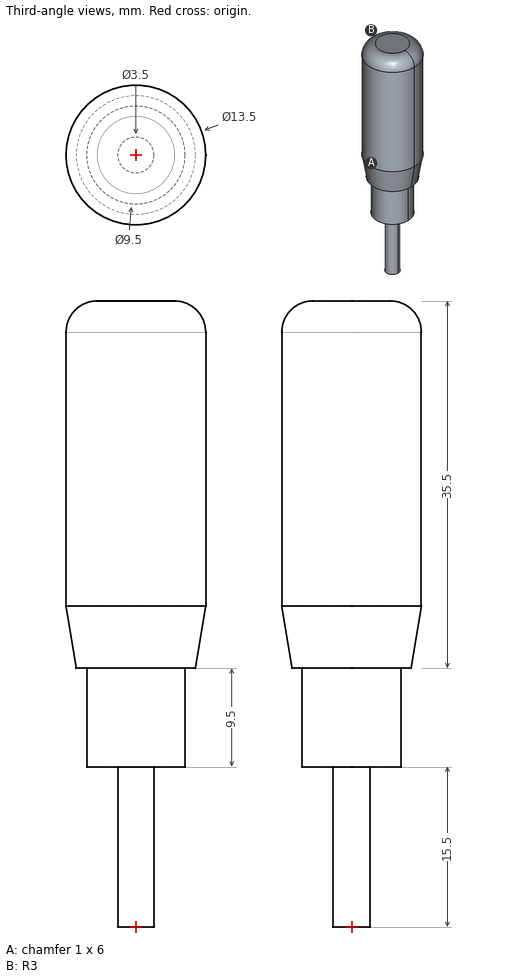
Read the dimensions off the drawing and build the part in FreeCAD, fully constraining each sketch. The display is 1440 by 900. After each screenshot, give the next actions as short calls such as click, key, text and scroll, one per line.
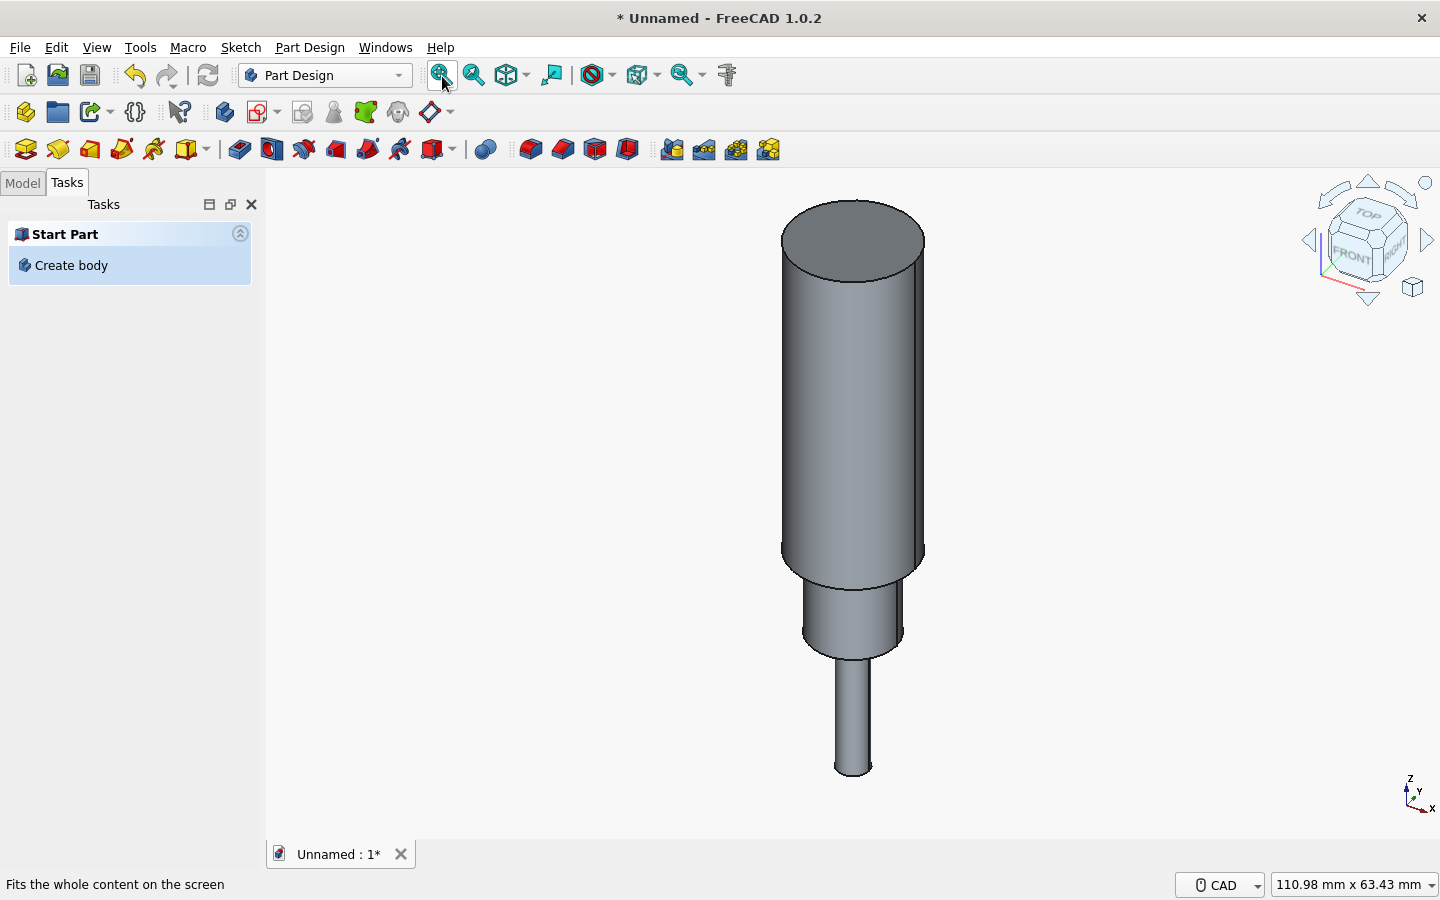
key(0)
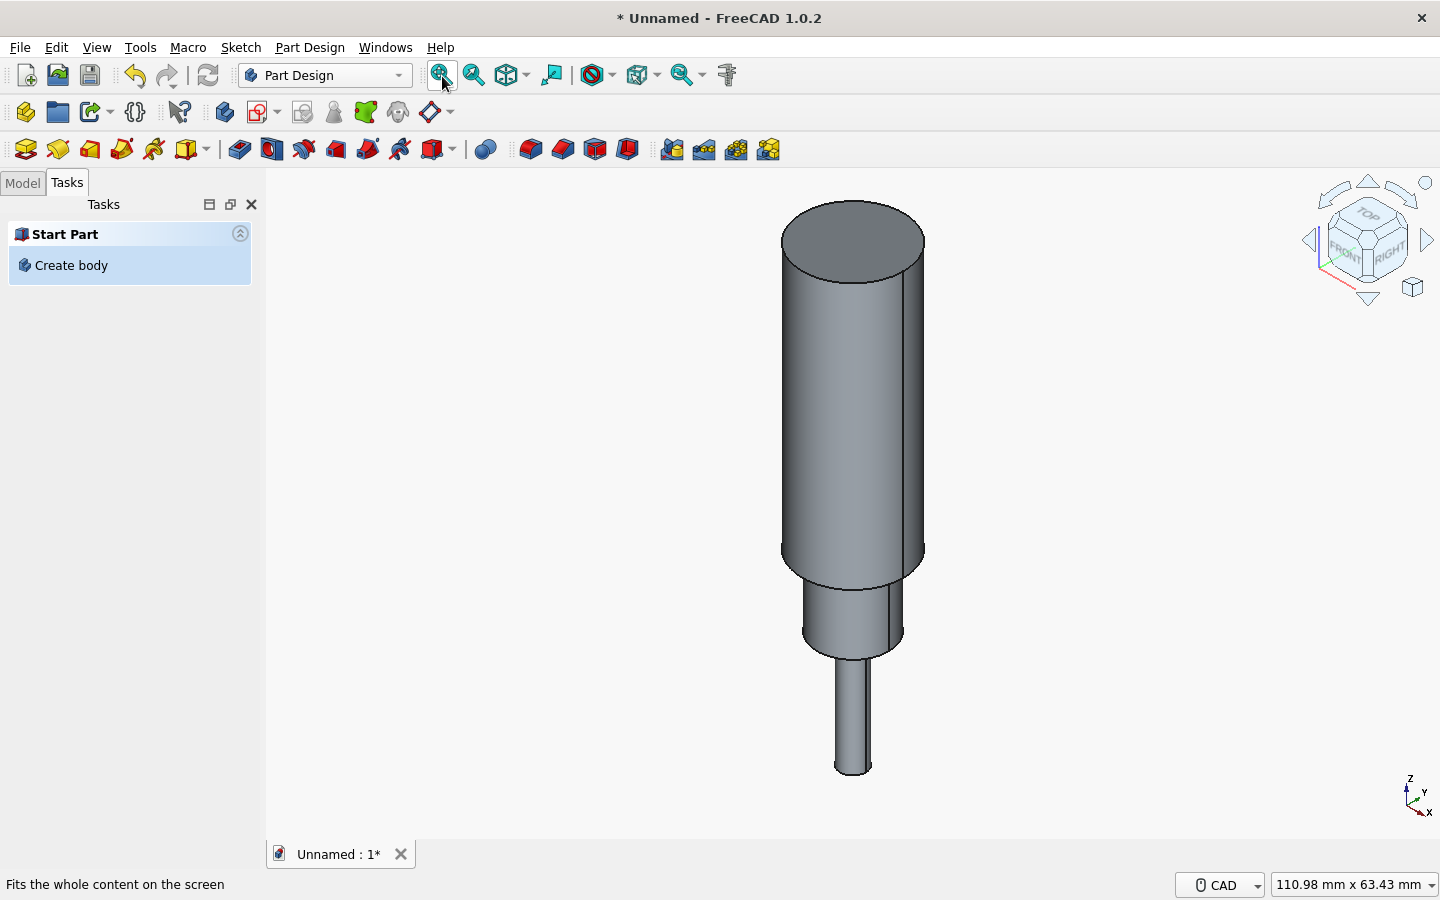
click(789, 567)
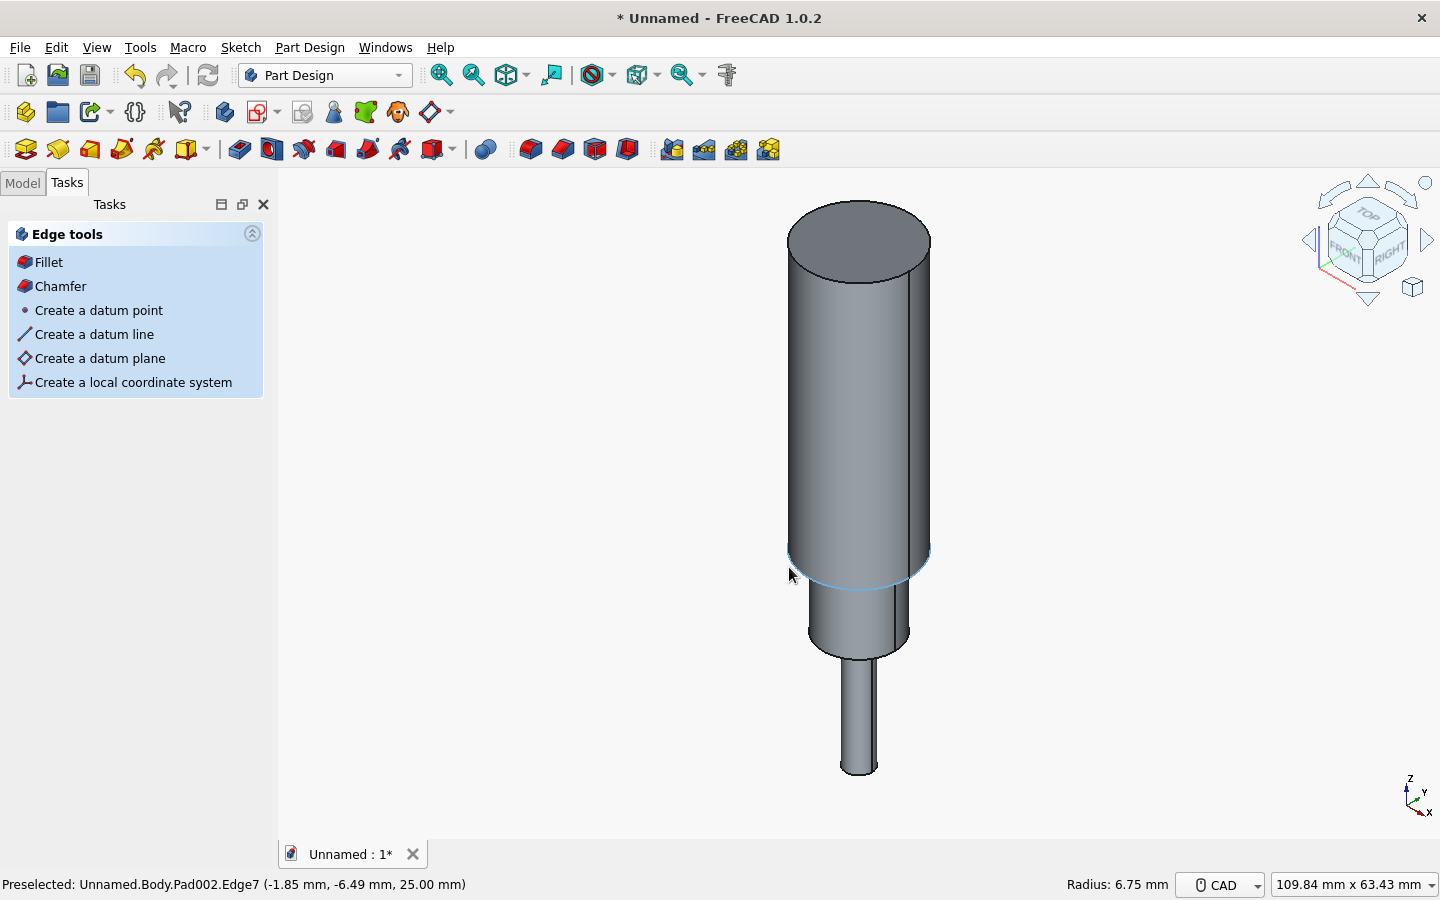
click(564, 150)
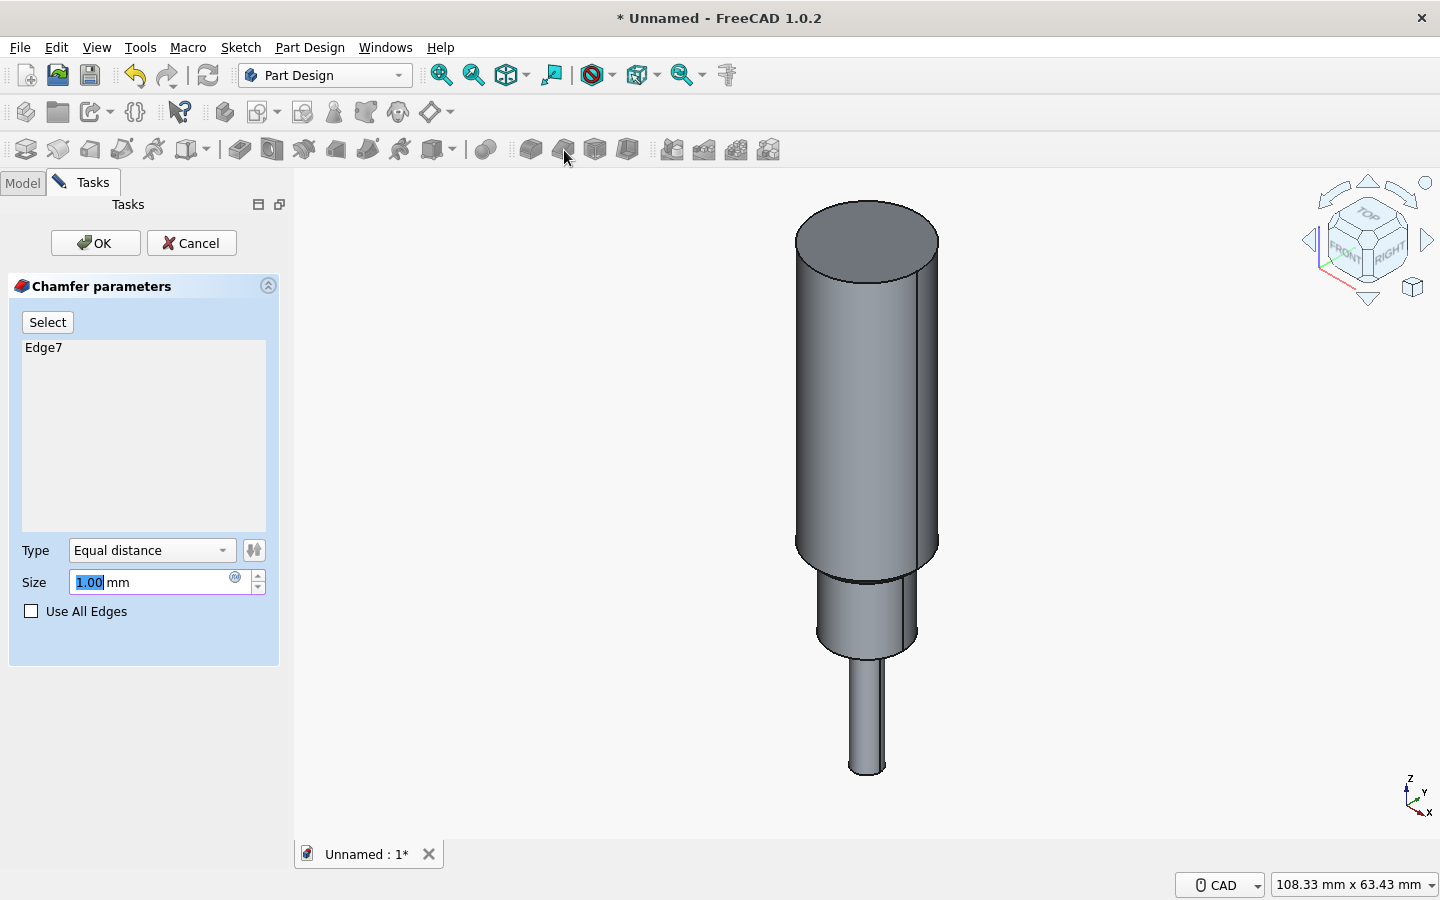
text(1)
key(Tab)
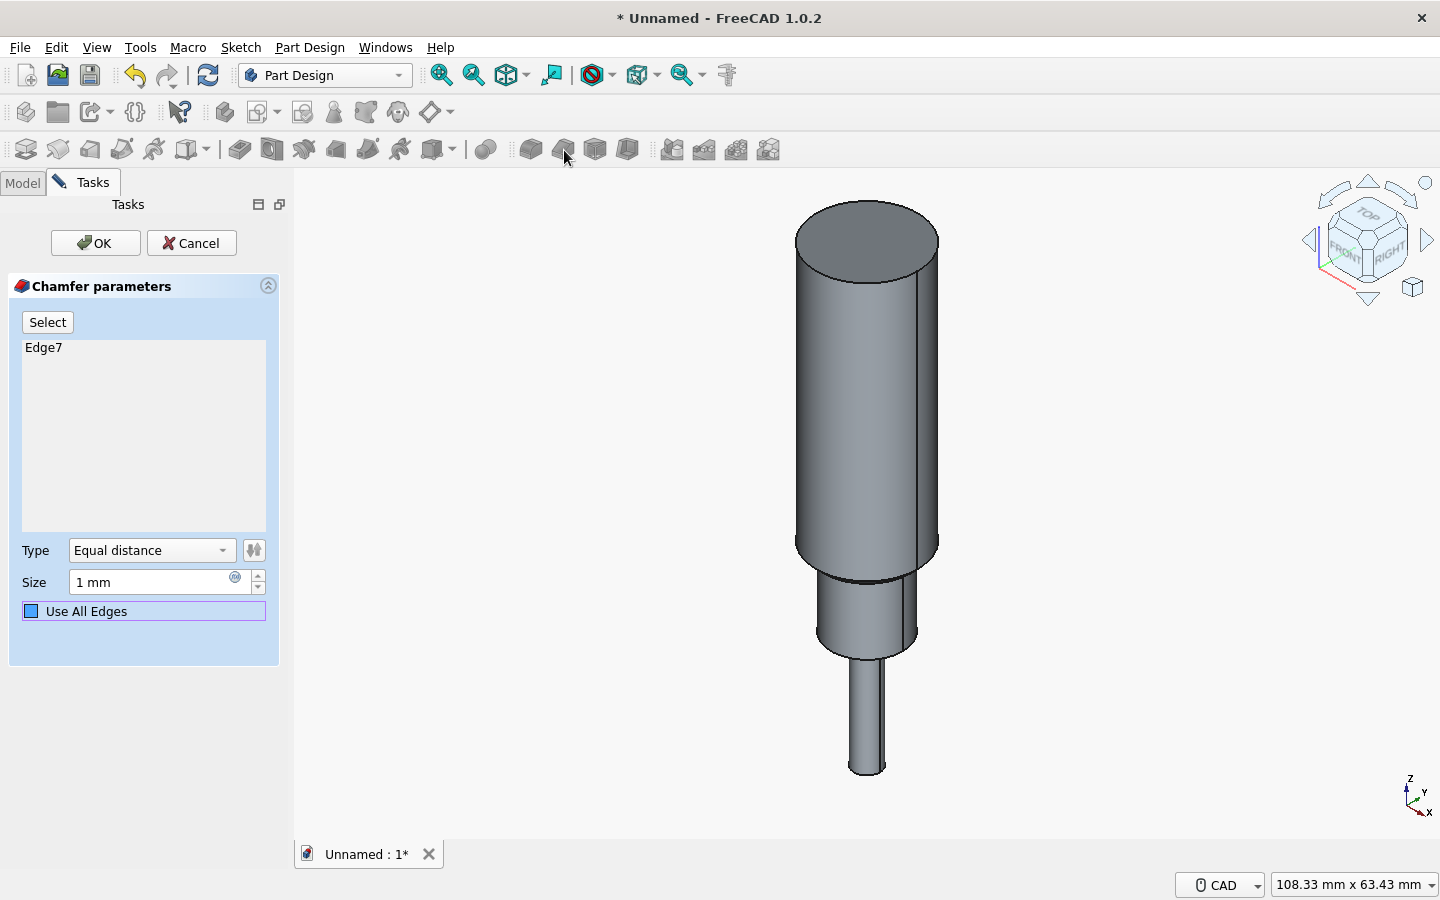
click(153, 550)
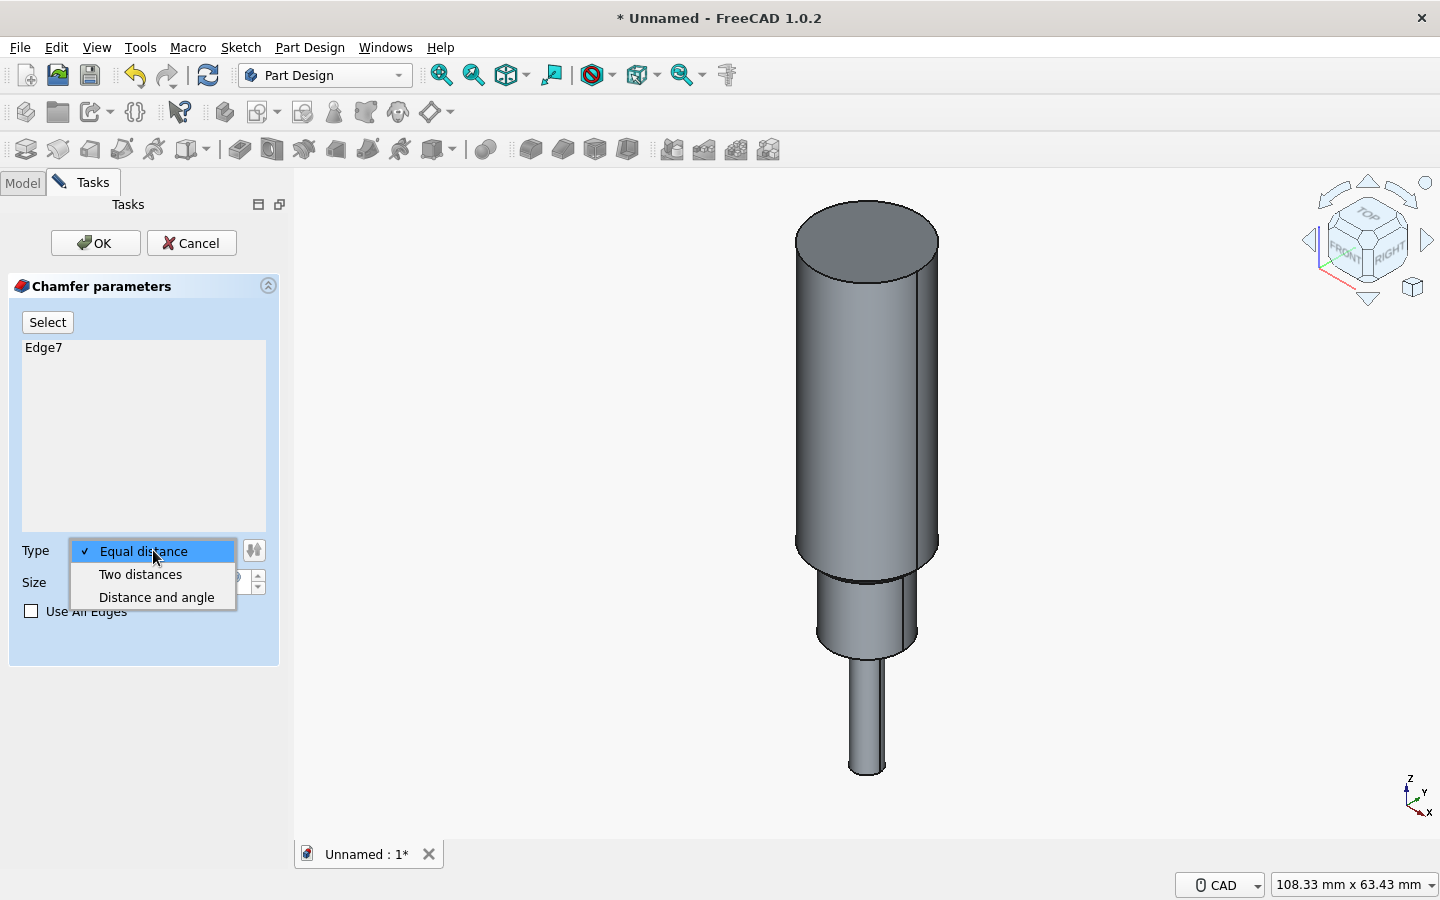
click(152, 574)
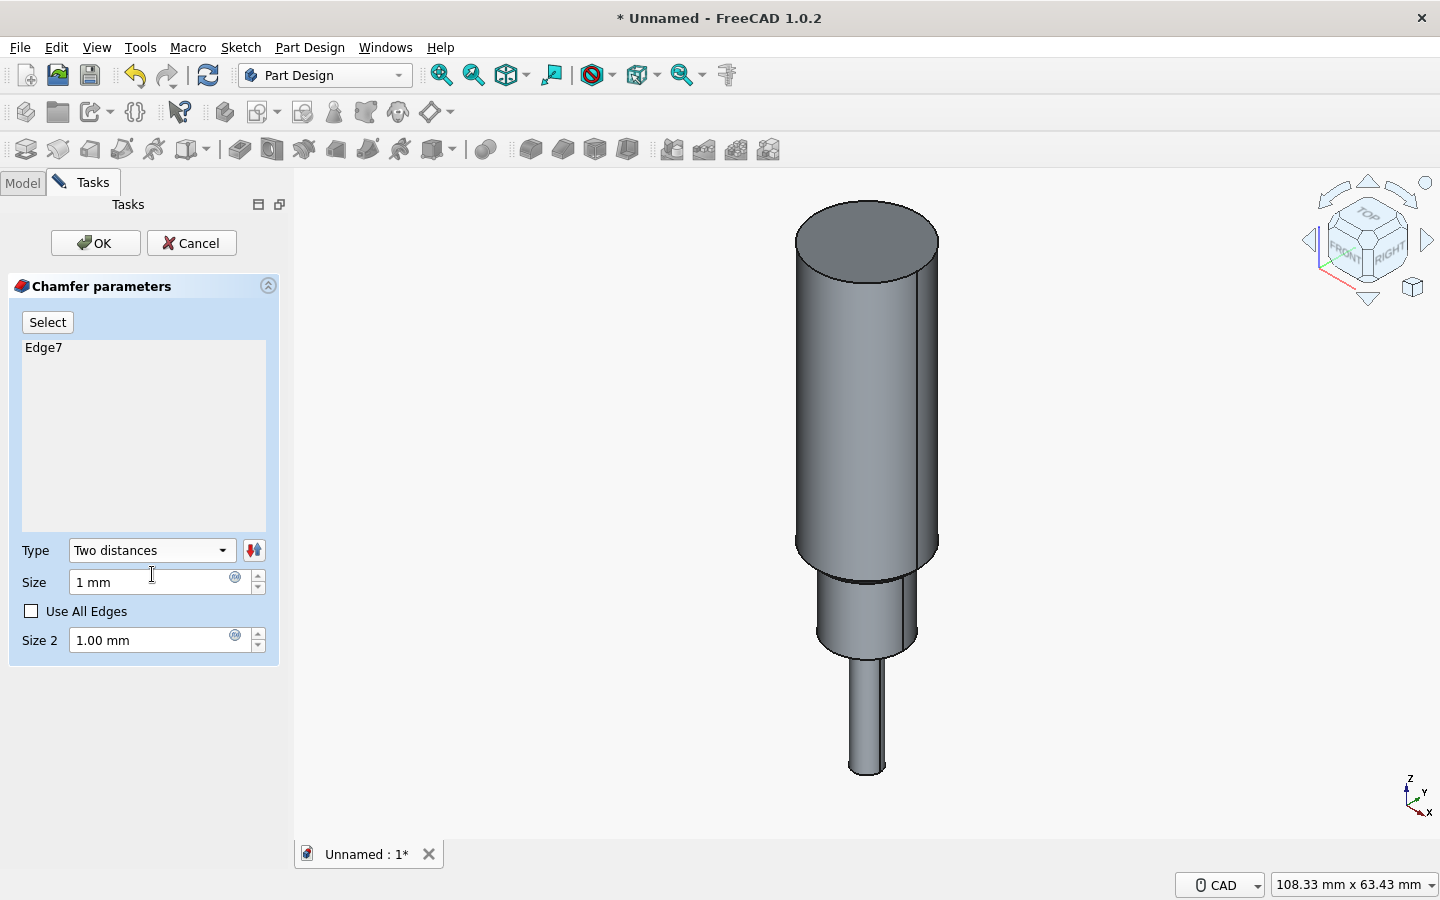
triple_click(160, 640)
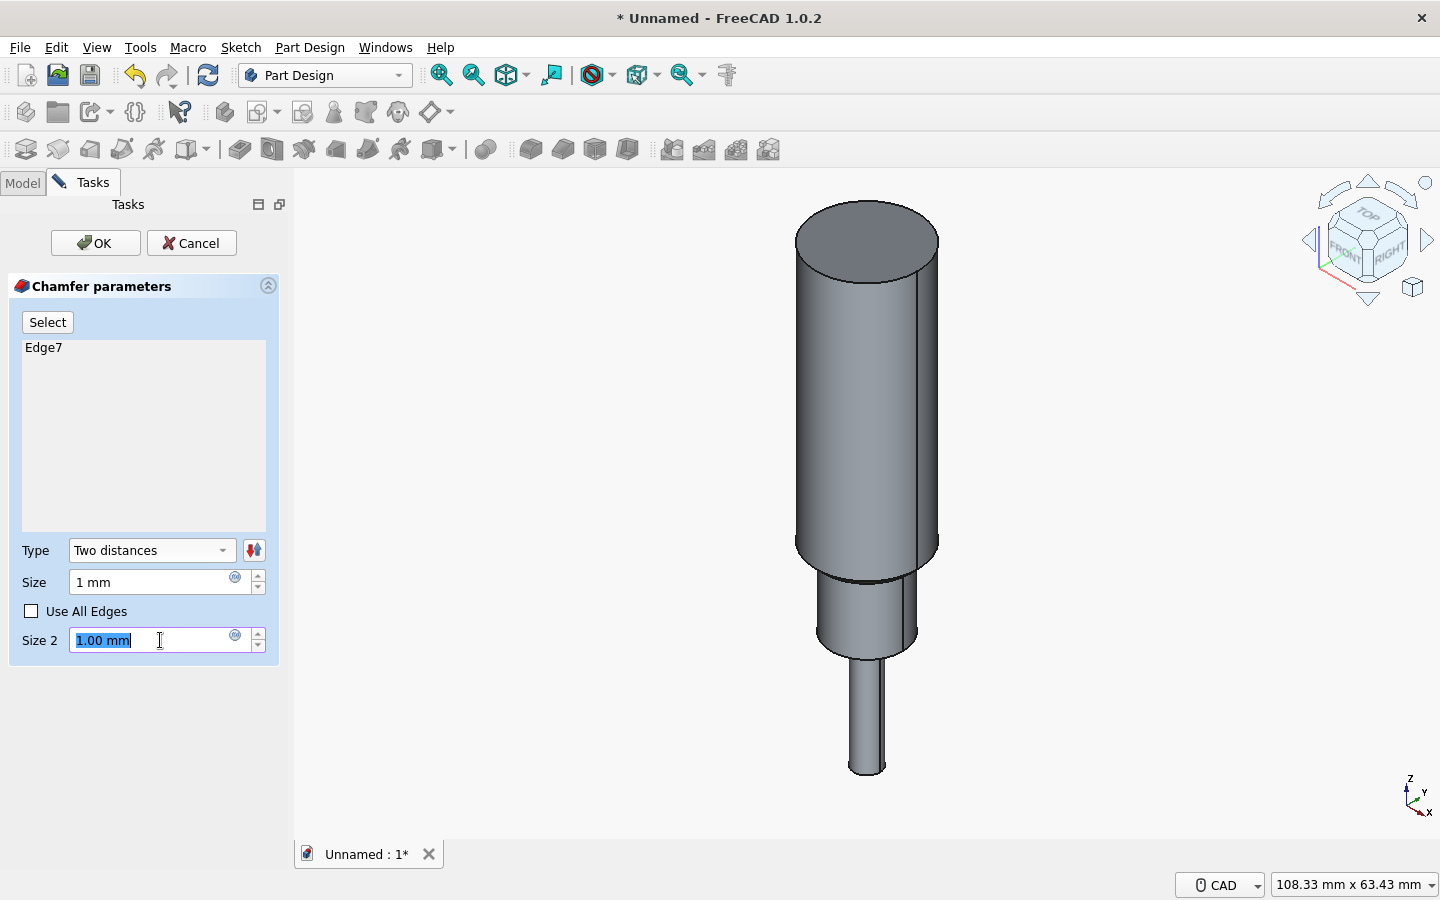
text(6)
key(Tab)